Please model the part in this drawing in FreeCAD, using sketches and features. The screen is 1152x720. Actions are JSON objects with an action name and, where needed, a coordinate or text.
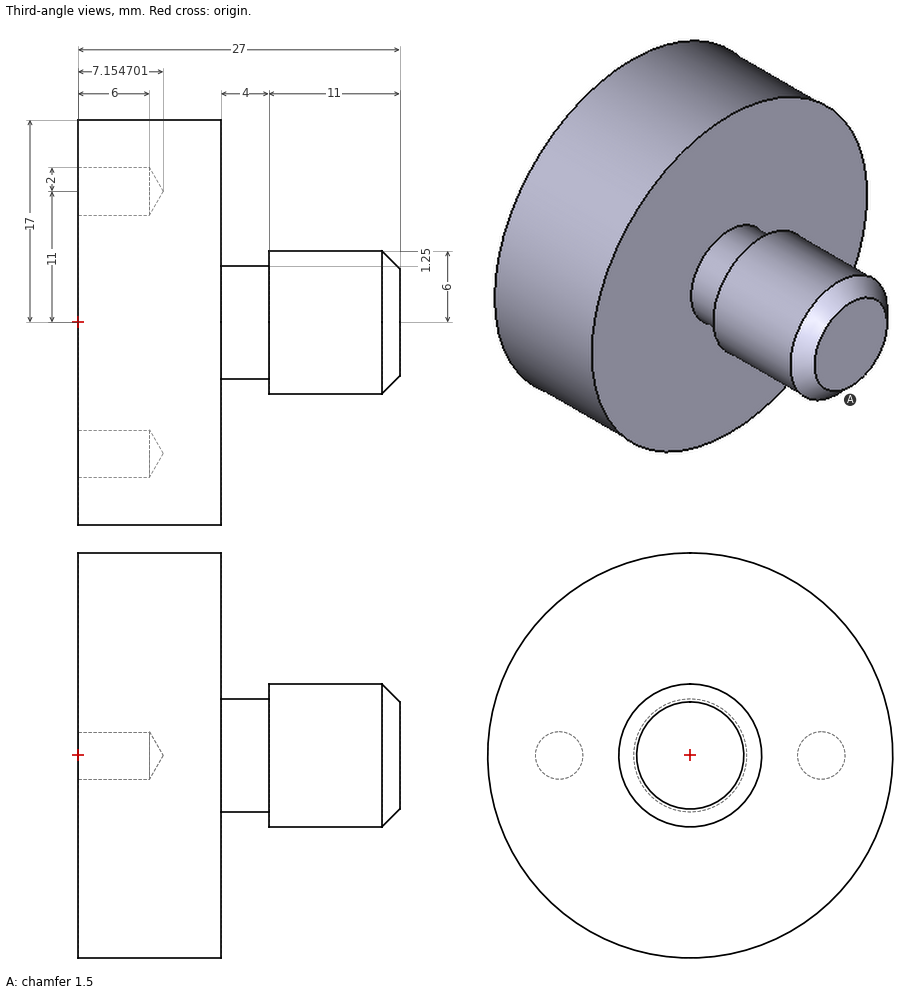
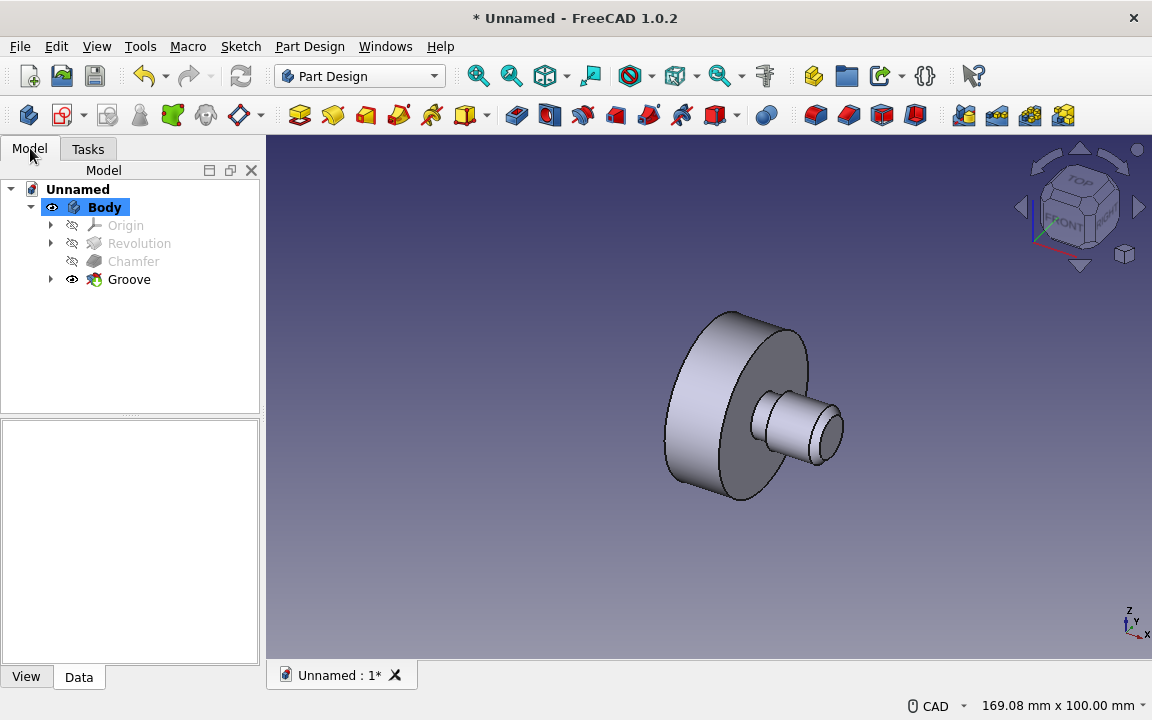
{"action": "left_click", "coordinate": [117, 279]}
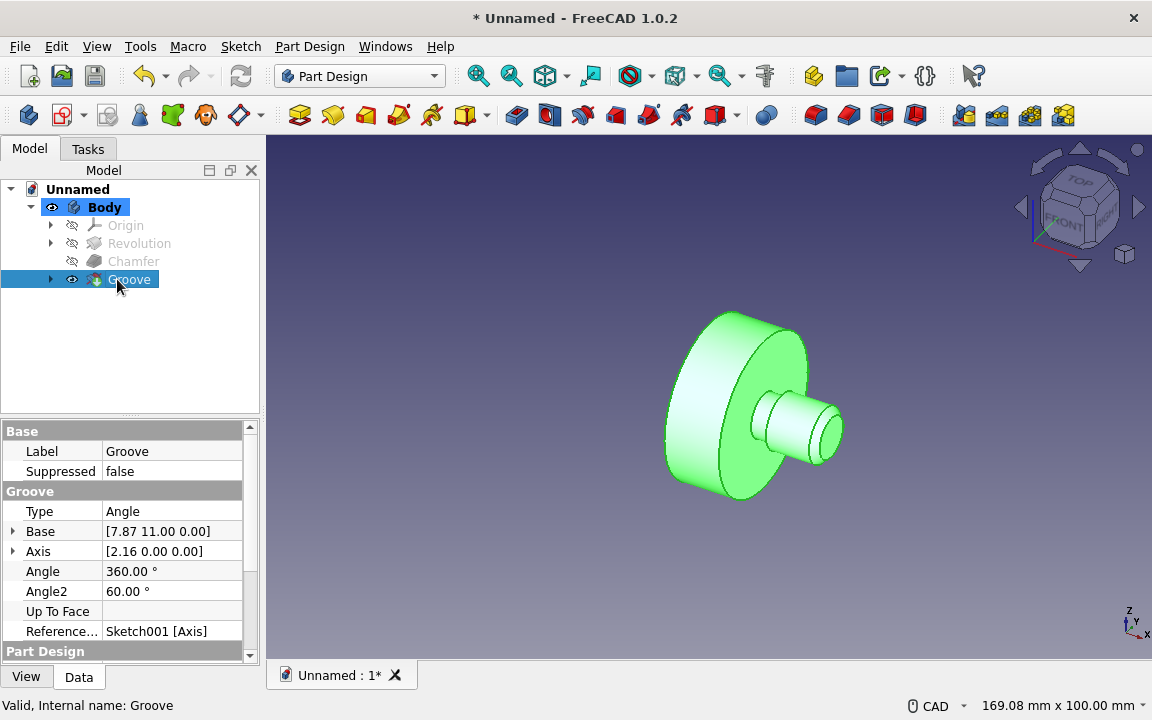
{"action": "left_click", "coordinate": [964, 116]}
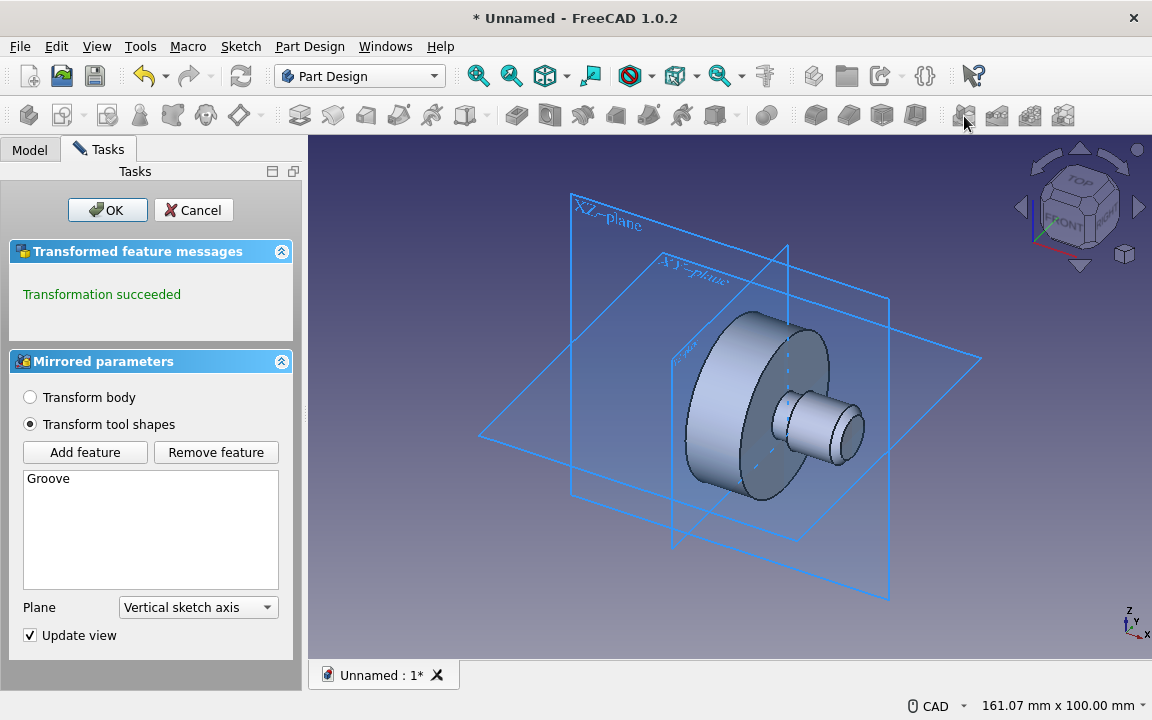
{"action": "left_click", "coordinate": [199, 608]}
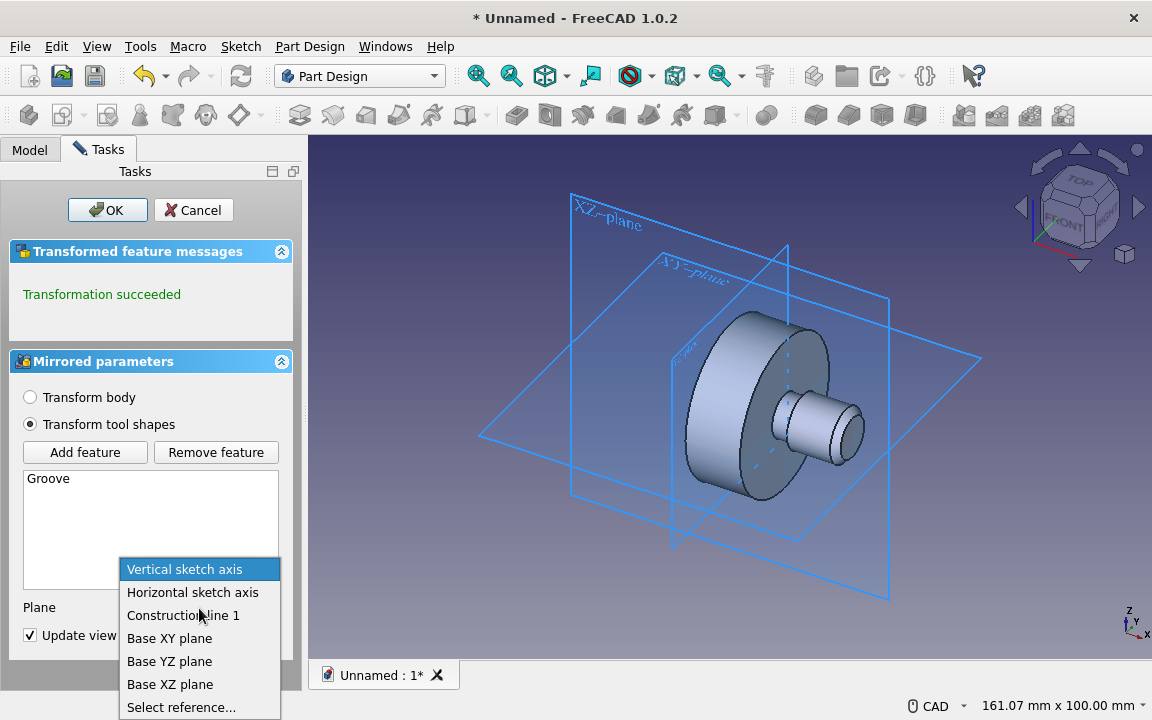
{"action": "left_click", "coordinate": [198, 684]}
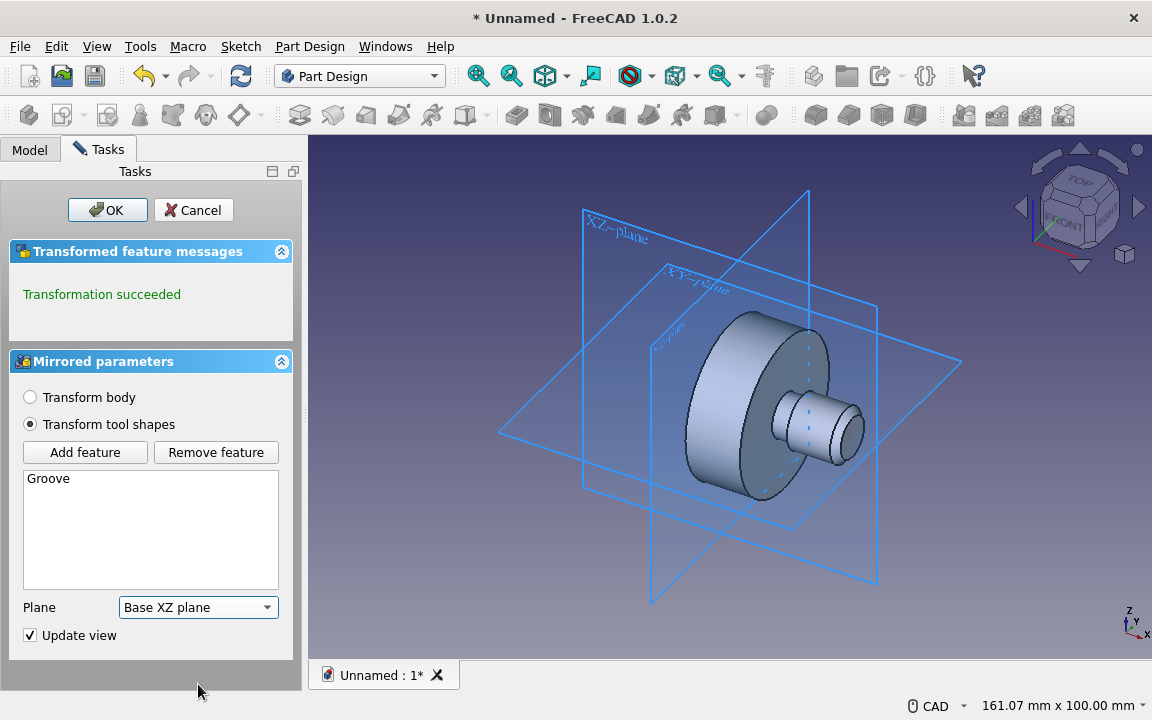
{"action": "left_click", "coordinate": [108, 210]}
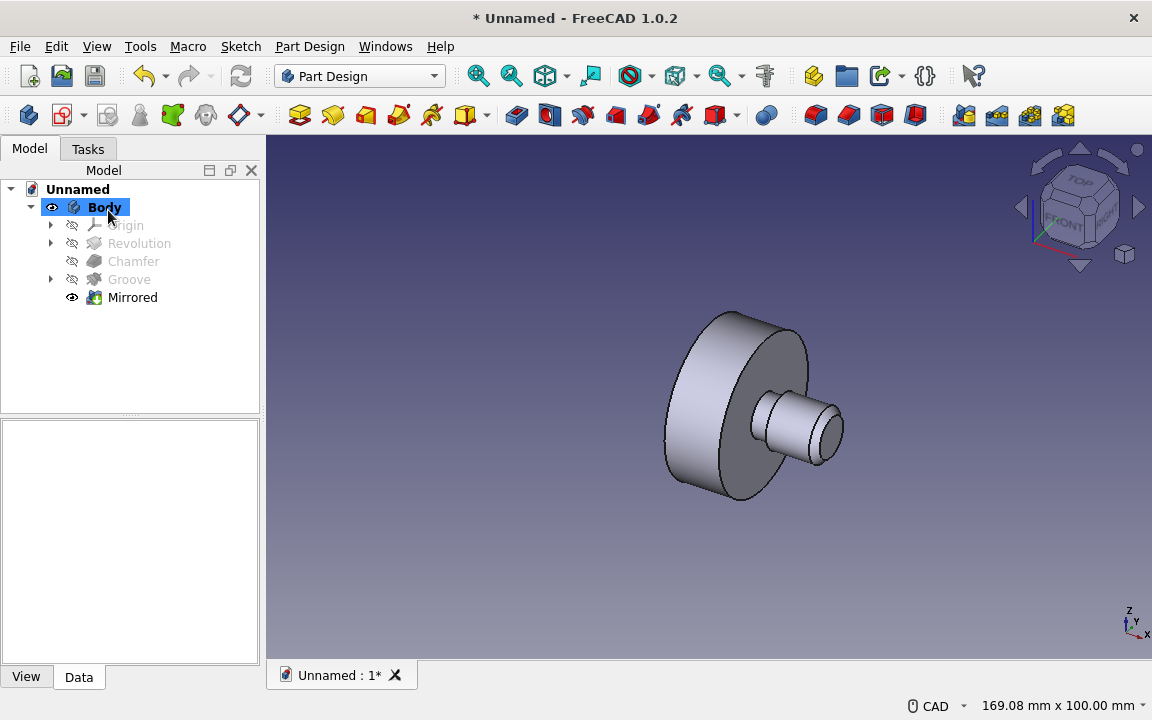
{"action": "key", "text": "0"}